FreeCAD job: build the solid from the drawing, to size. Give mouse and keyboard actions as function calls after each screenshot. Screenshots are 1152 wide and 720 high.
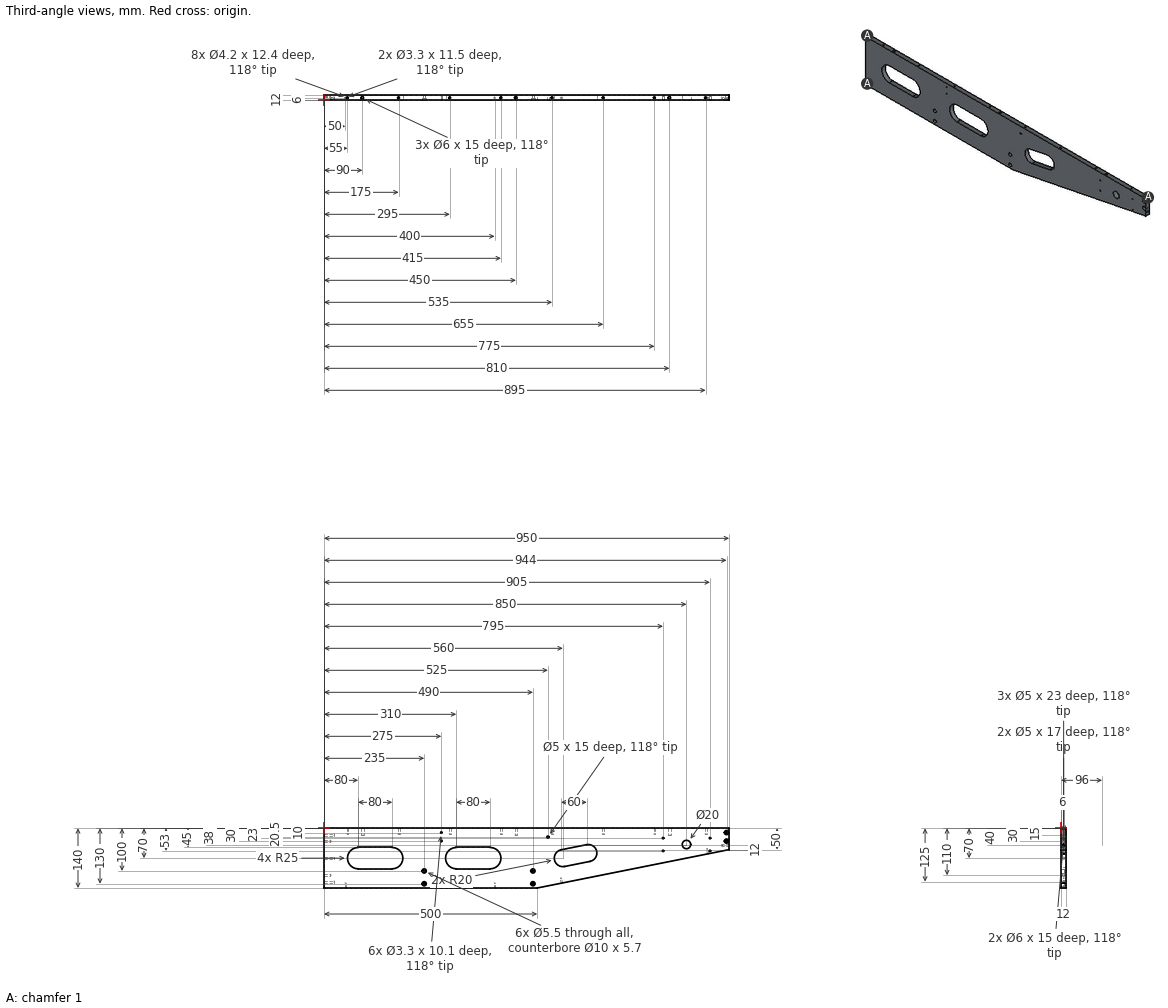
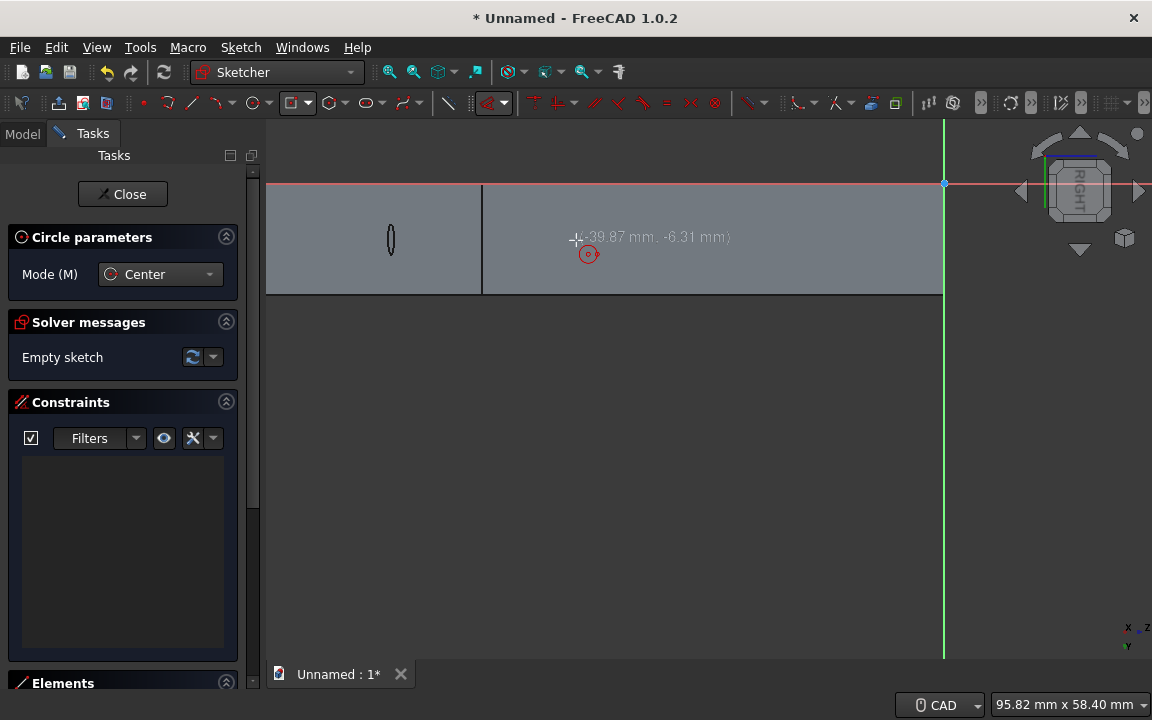
click(574, 239)
move(591, 223)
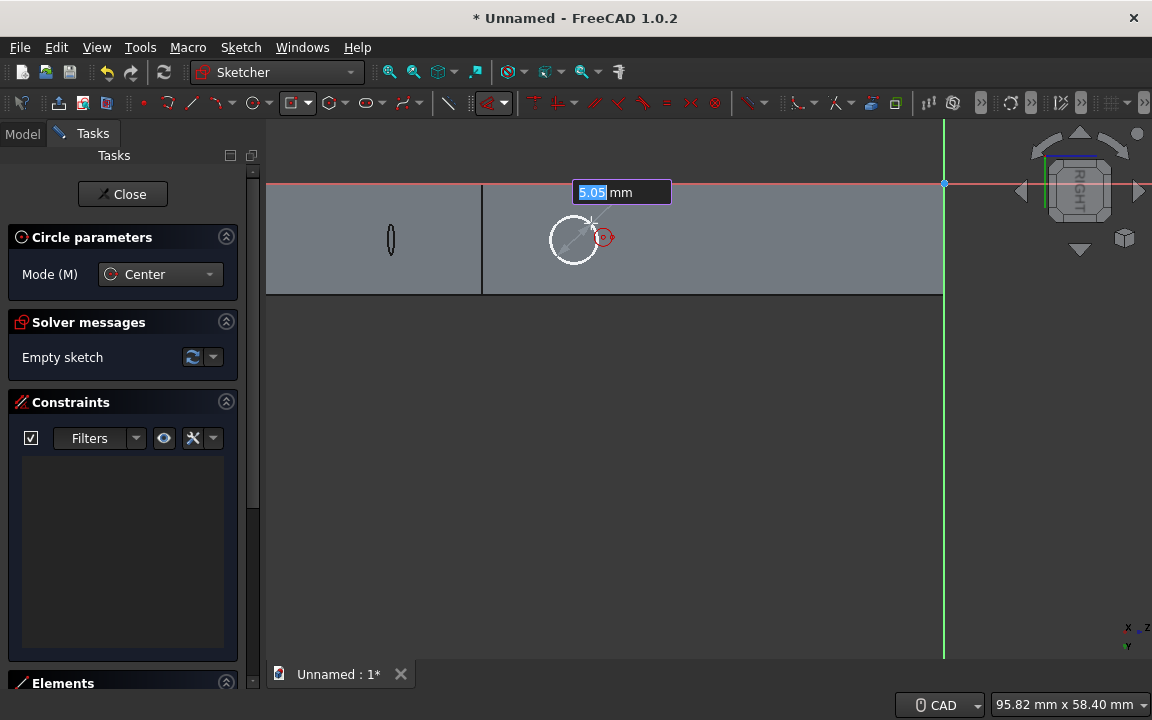
text(5)
key(Return)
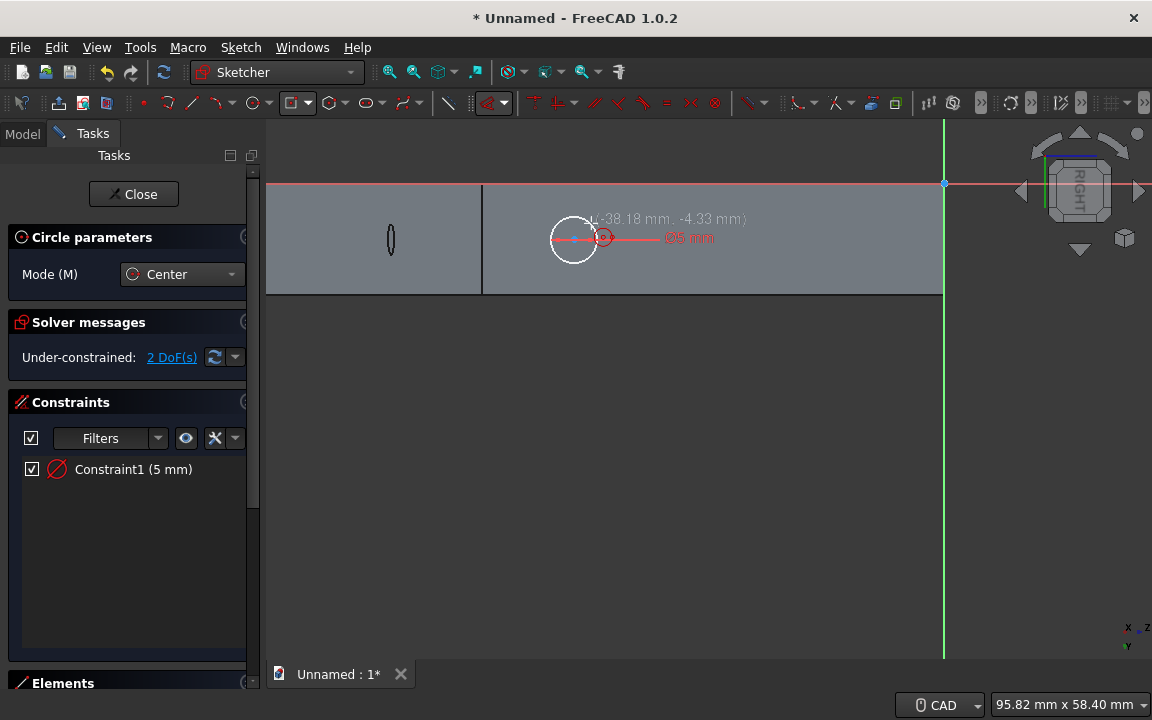
scroll(578, 243, down, 5)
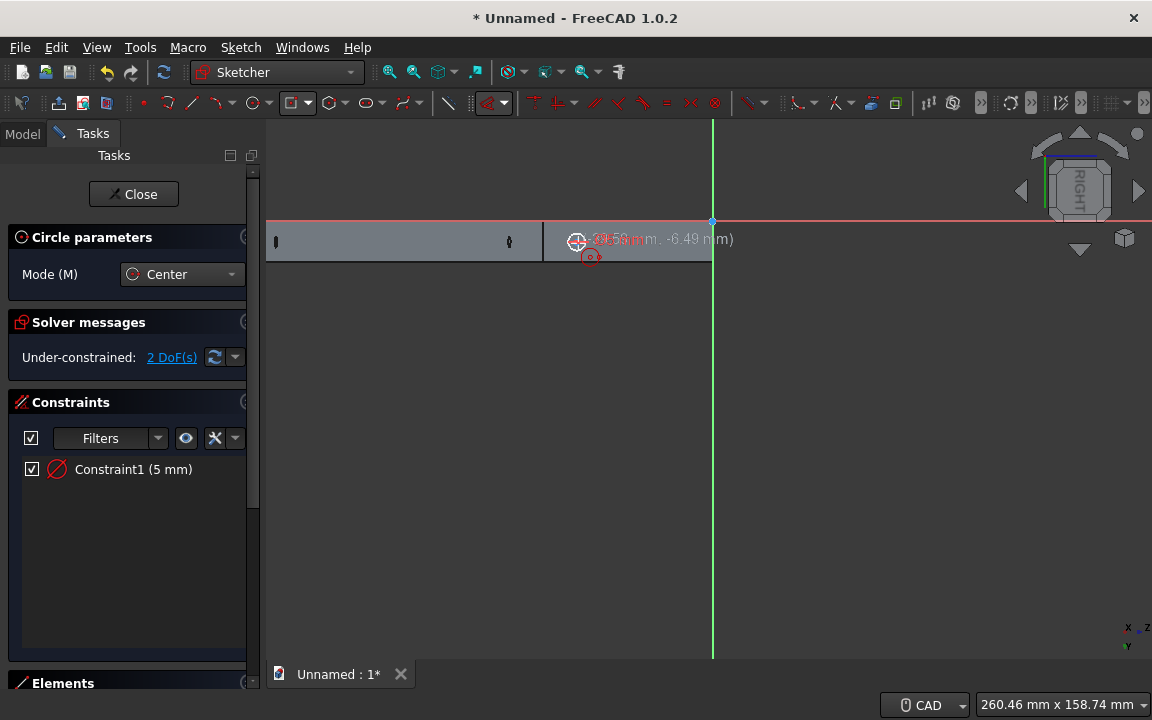
scroll(577, 548, up, 5)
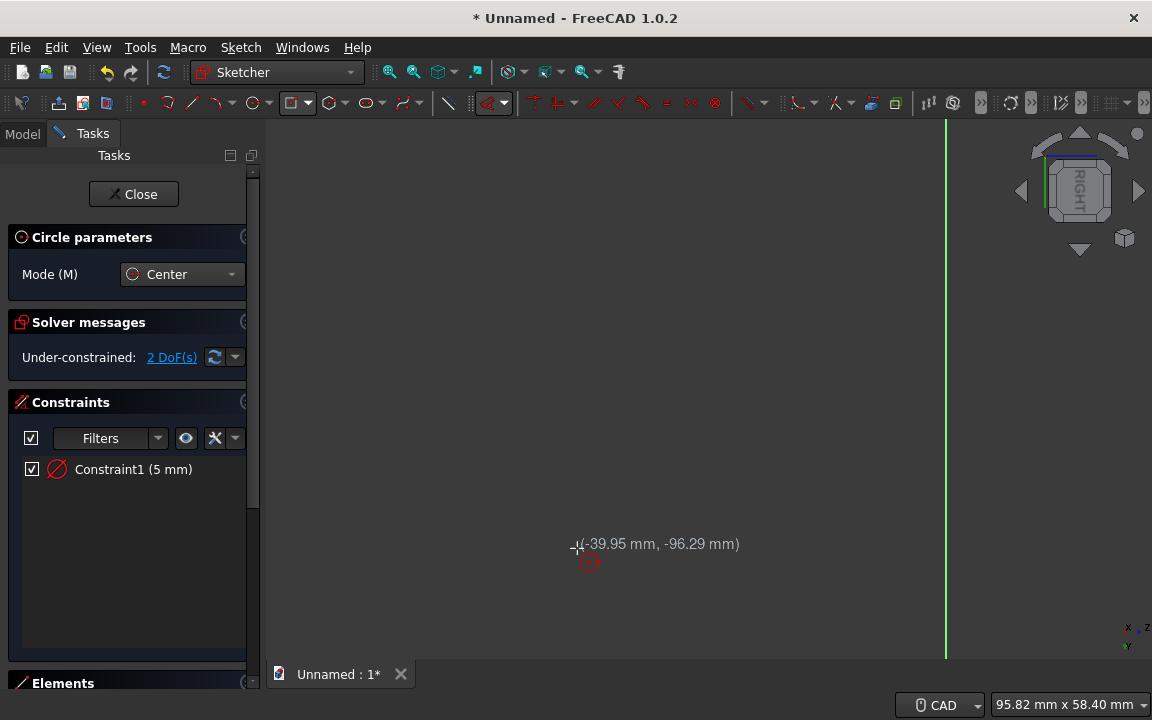
click(576, 547)
move(592, 530)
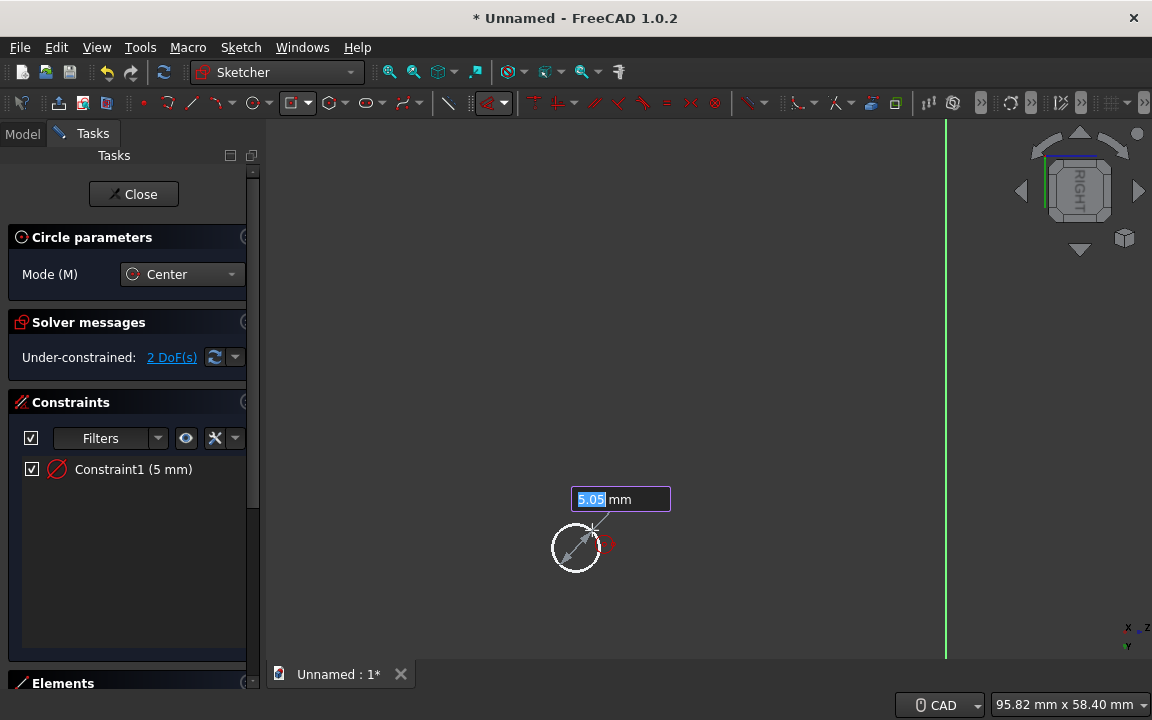
text(5)
key(Return)
key(Escape)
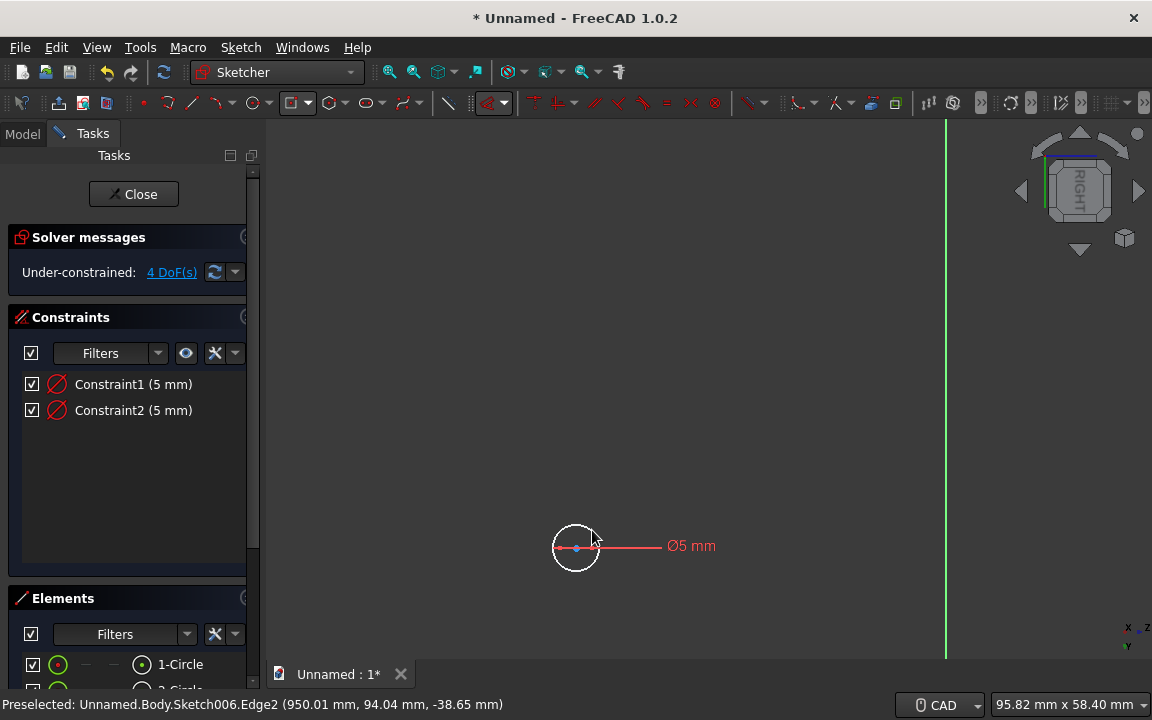
scroll(577, 549, down, 5)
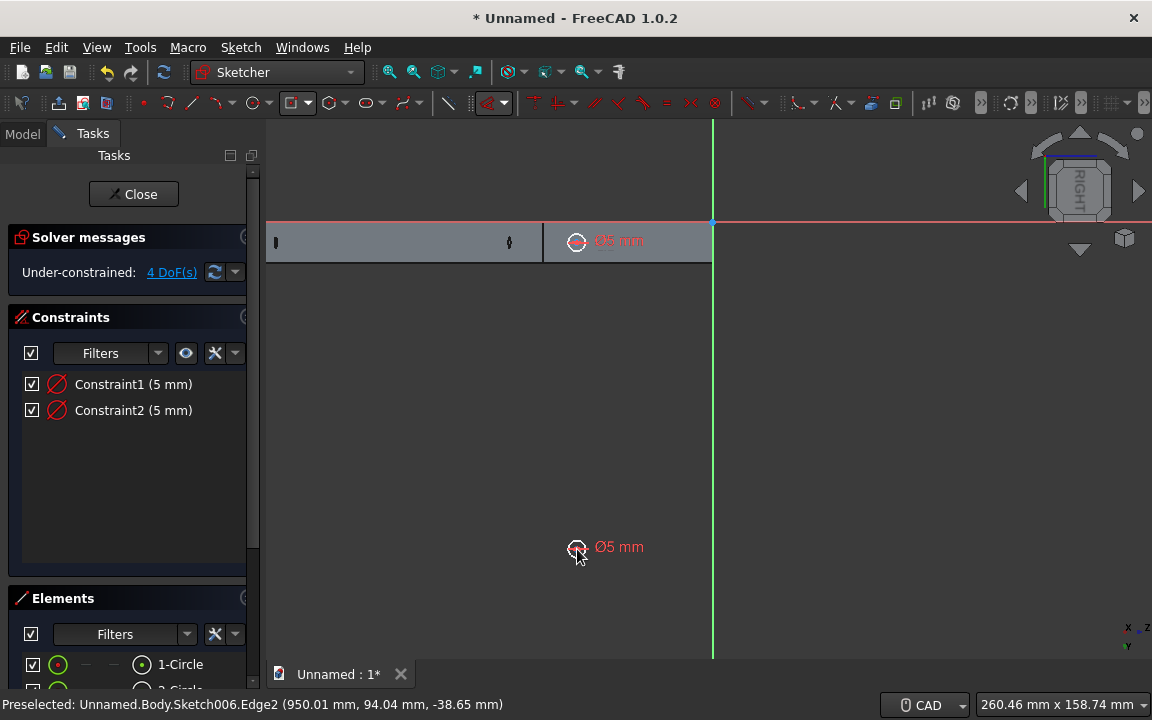
click(577, 243)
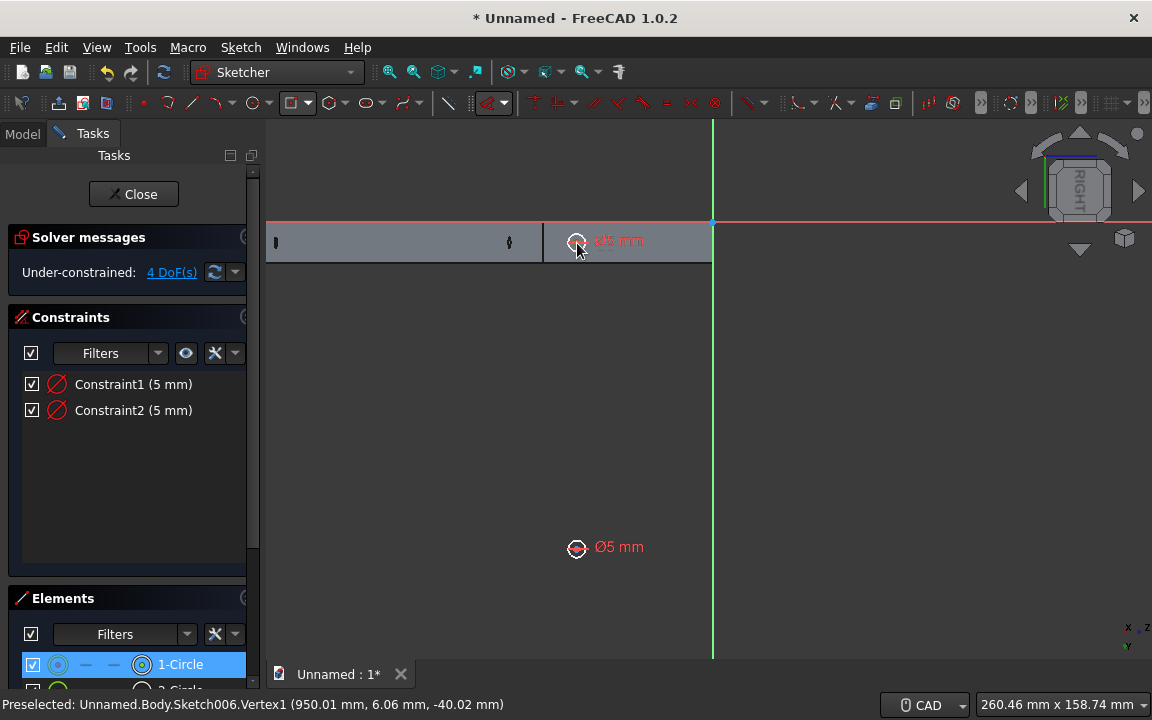
click(577, 549)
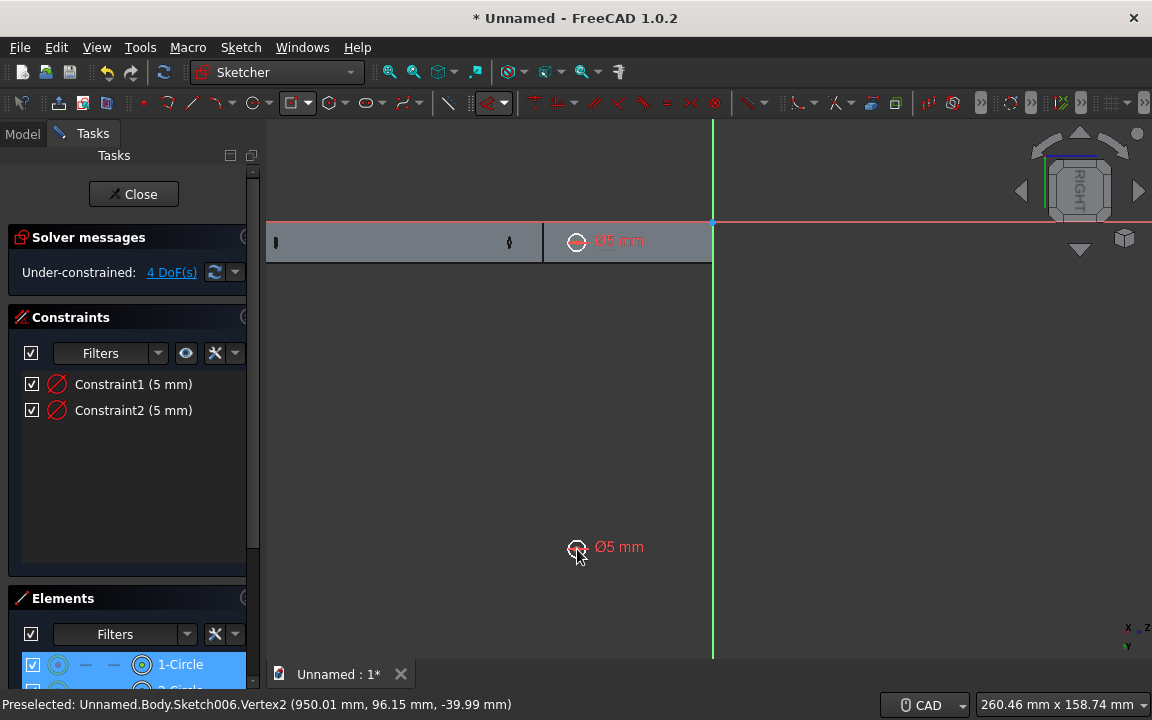
key(v)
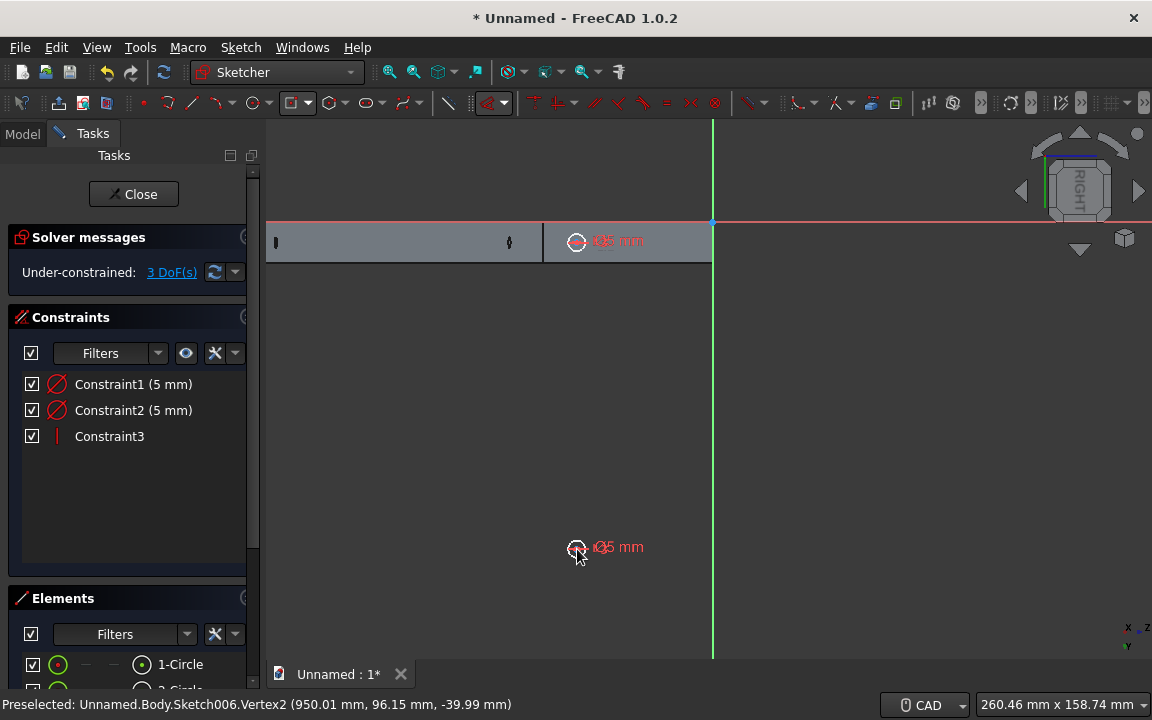
scroll(577, 243, up, 4)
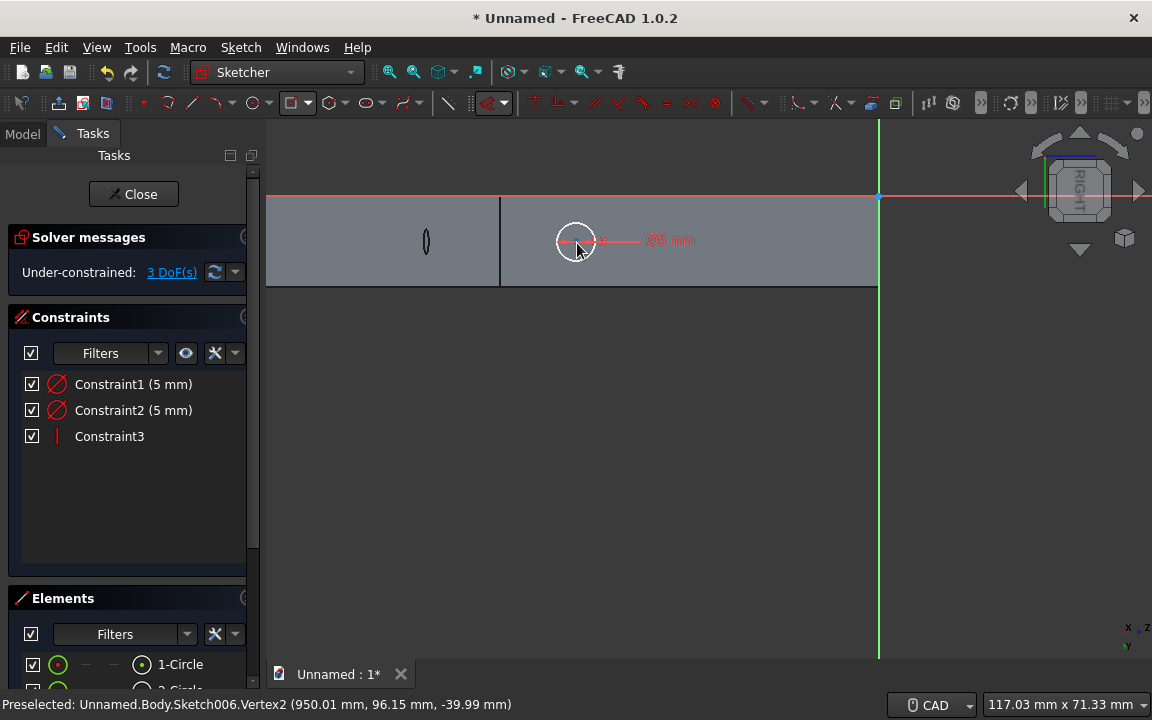
click(576, 242)